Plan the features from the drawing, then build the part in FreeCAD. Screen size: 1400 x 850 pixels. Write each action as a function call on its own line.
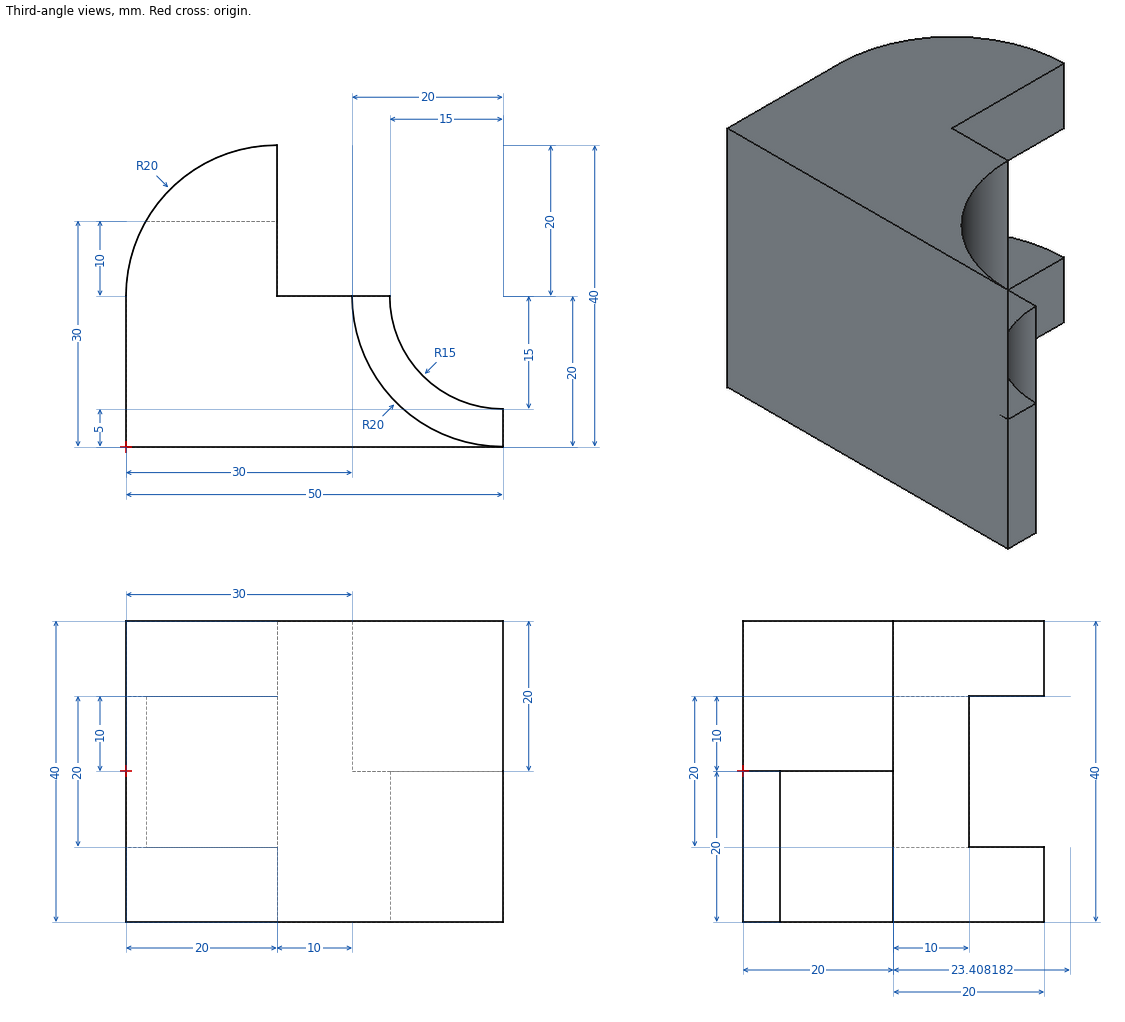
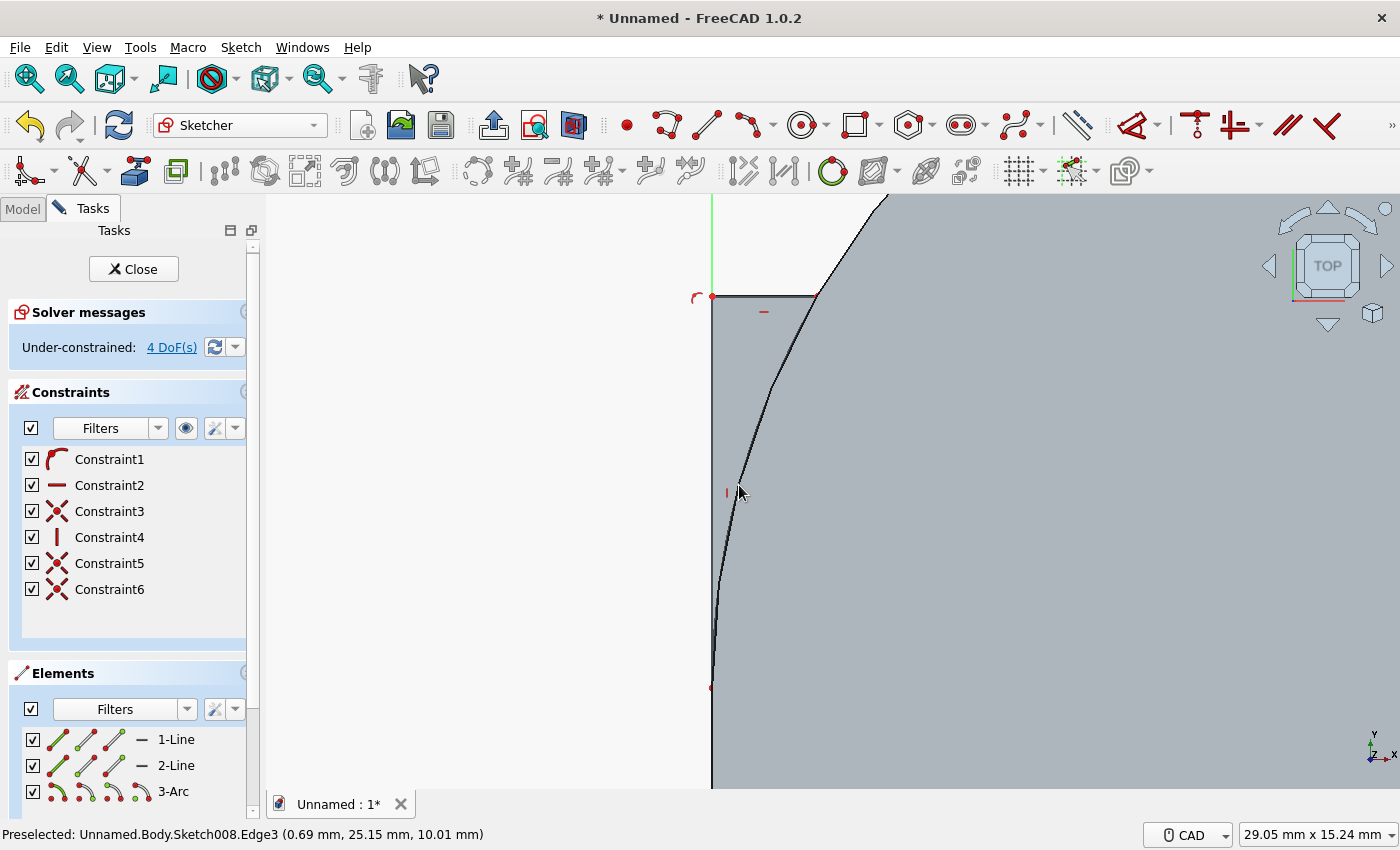
click(712, 414)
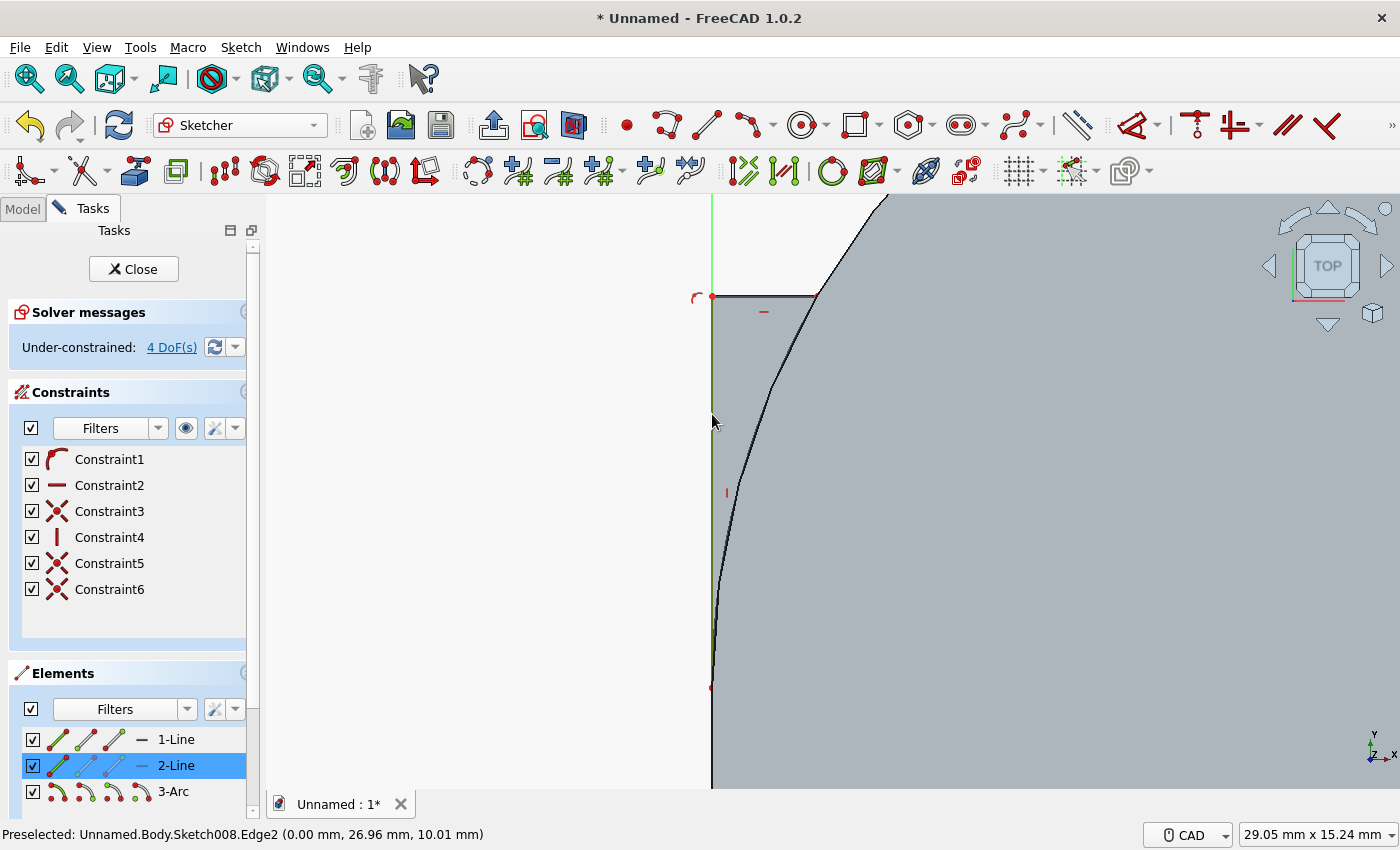
click(764, 408)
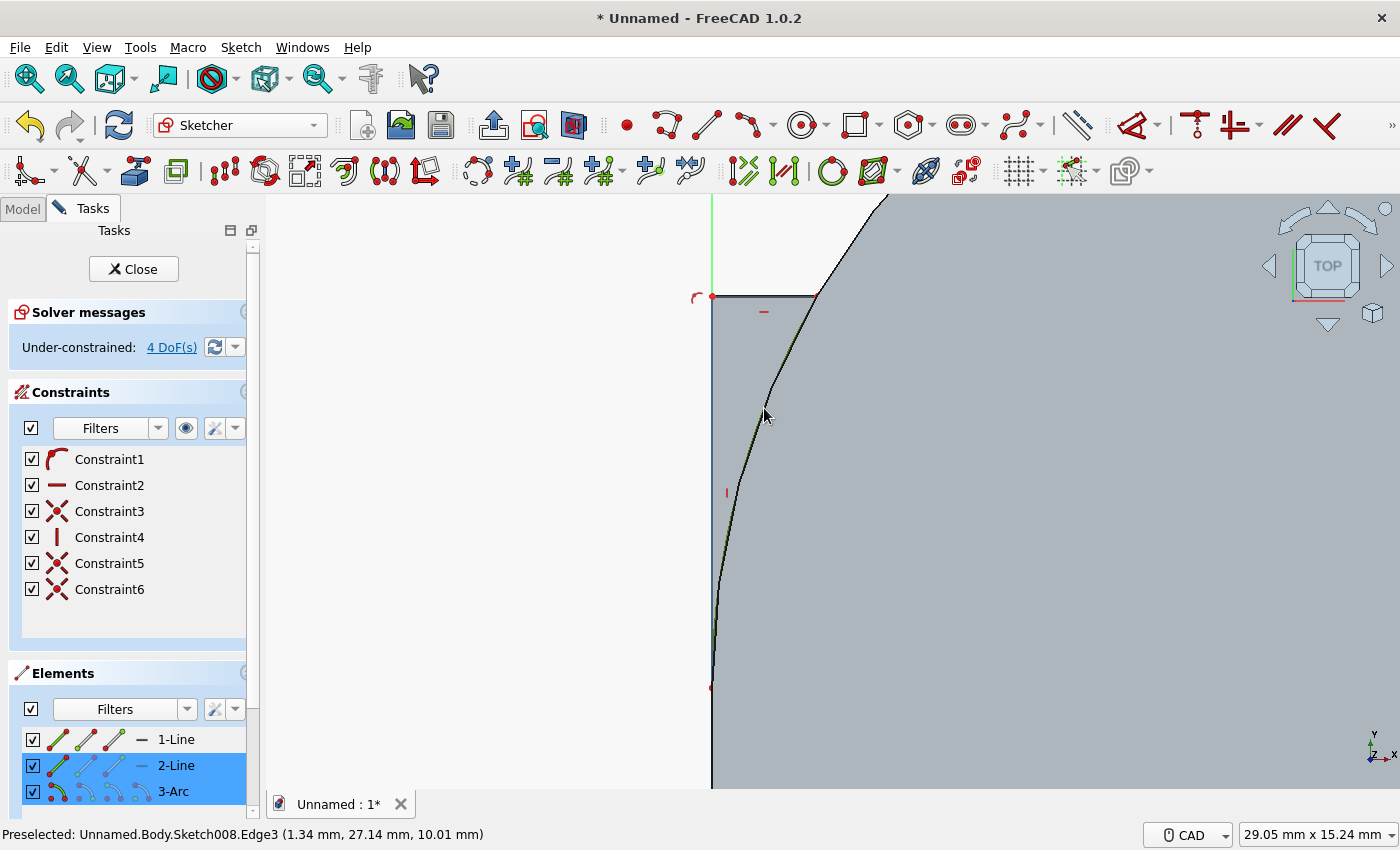
key(t)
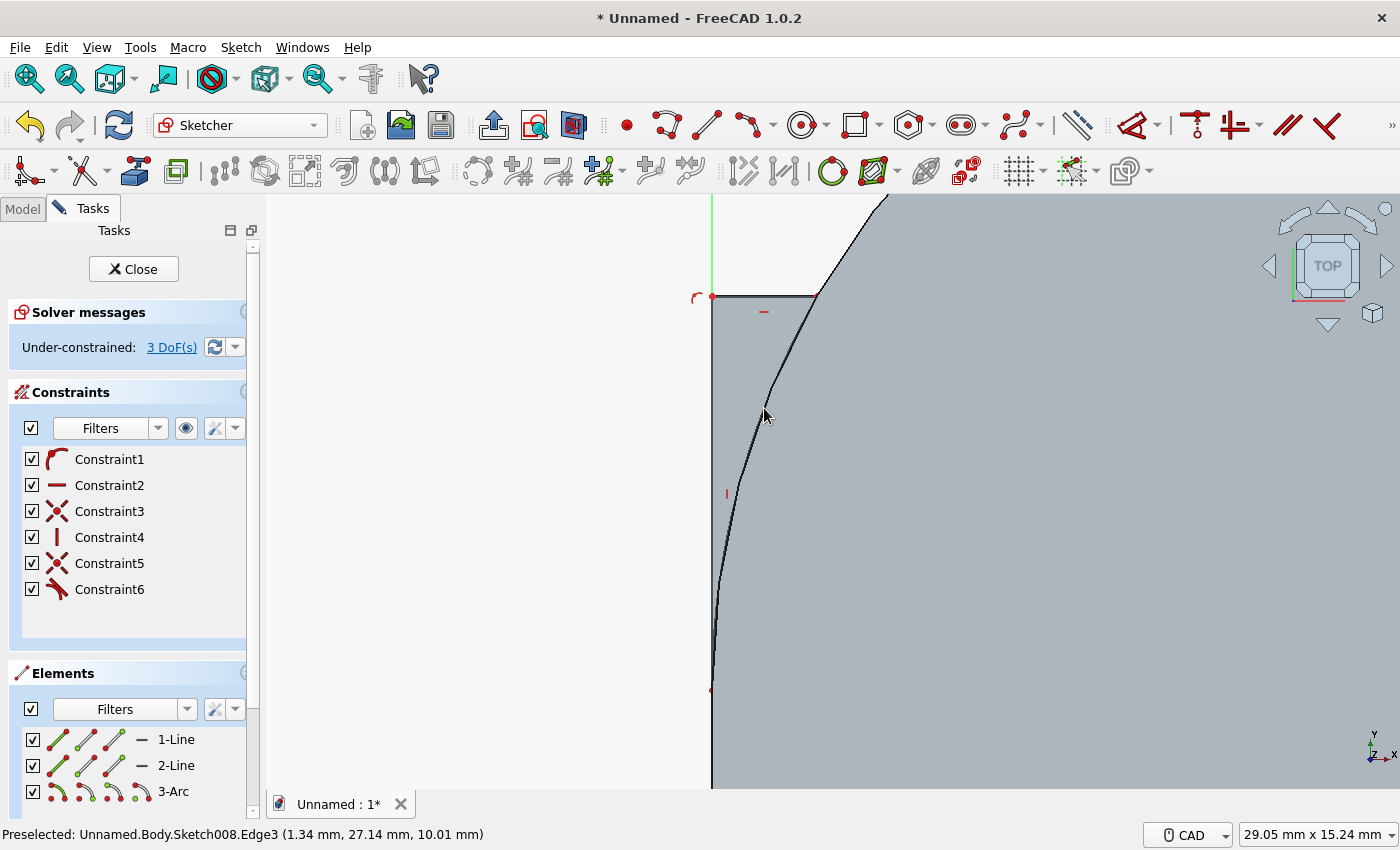
click(1132, 126)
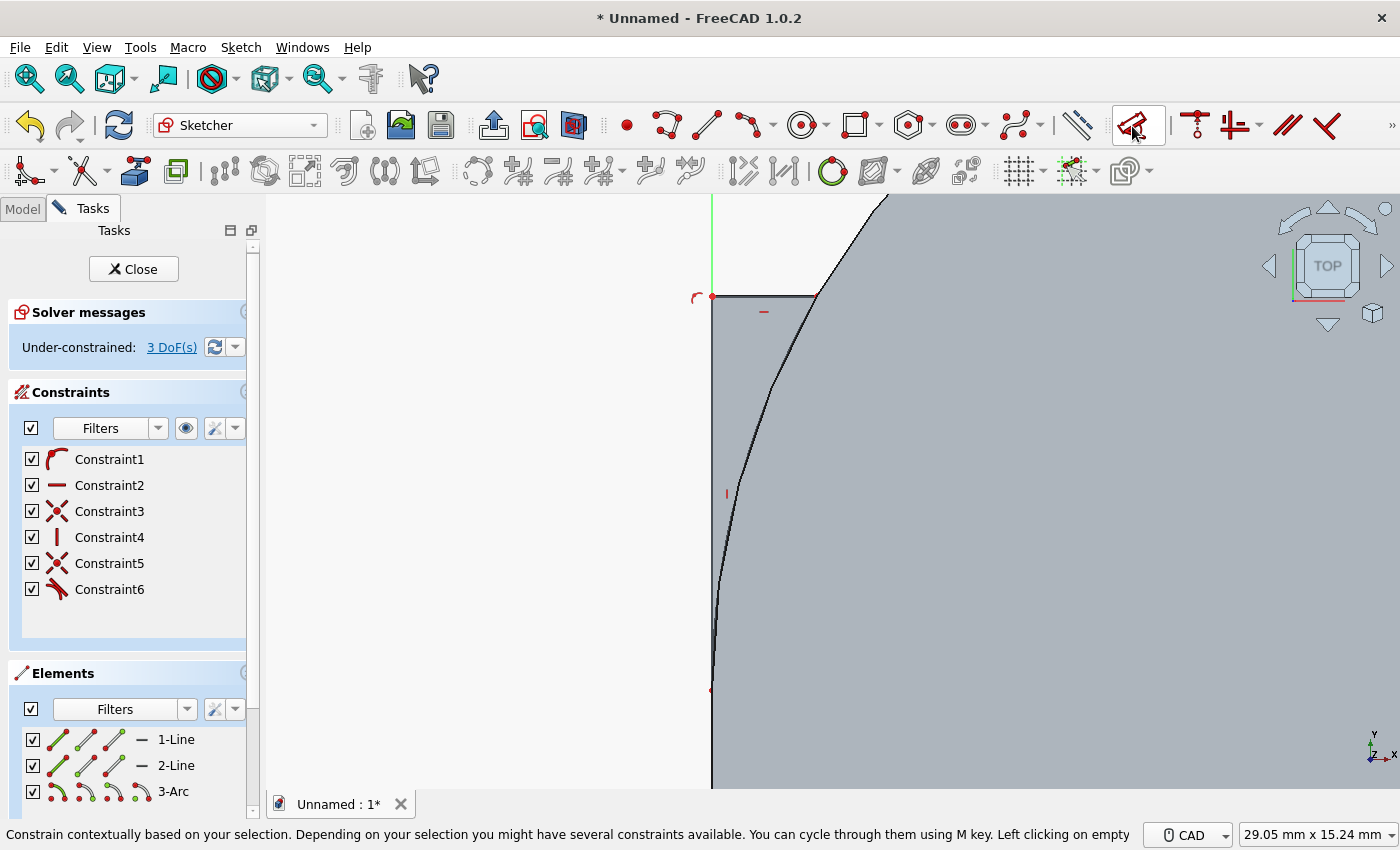
click(764, 408)
click(734, 397)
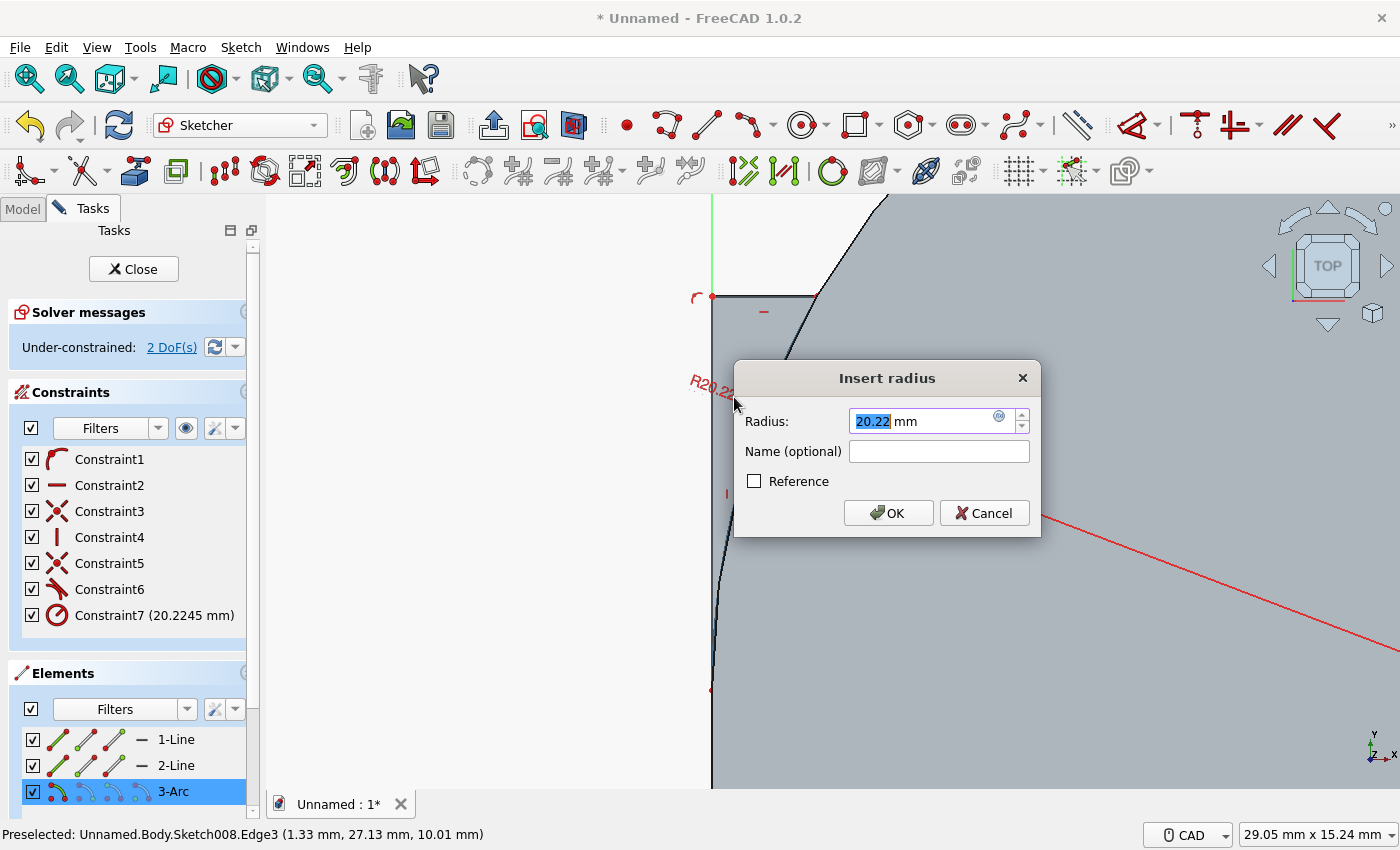
text(20)
key(Return)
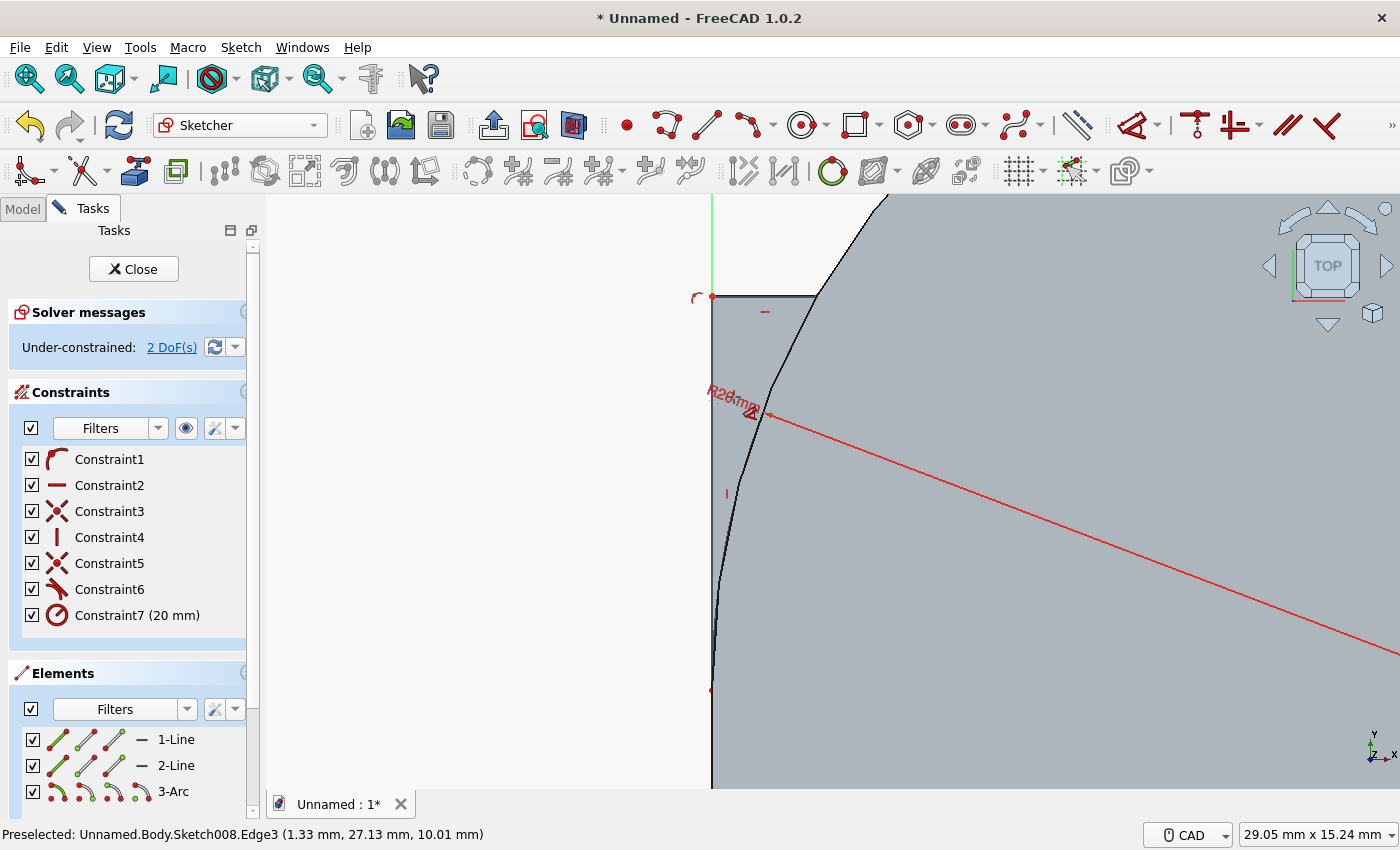
click(712, 415)
click(678, 494)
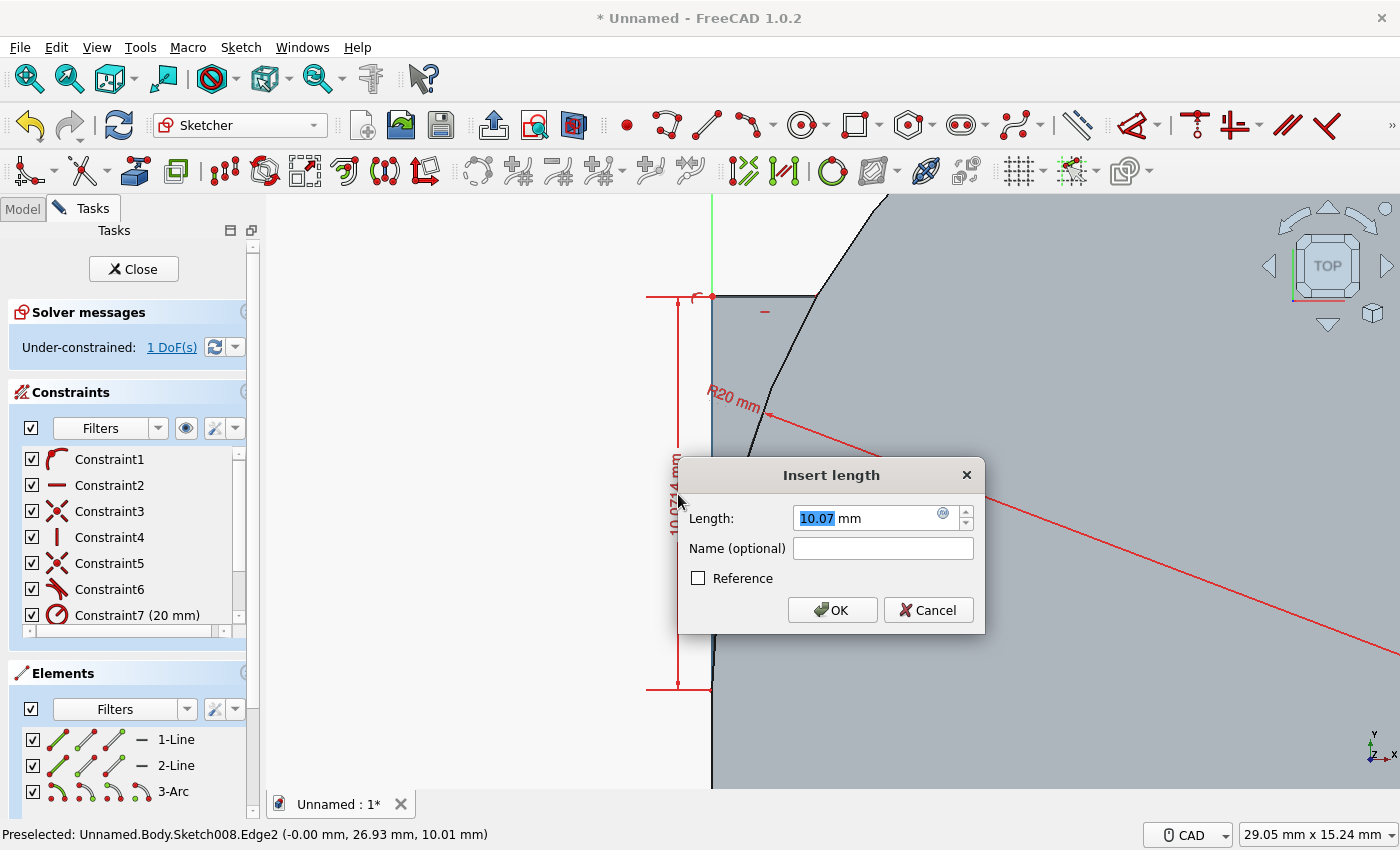
text(10)
key(Return)